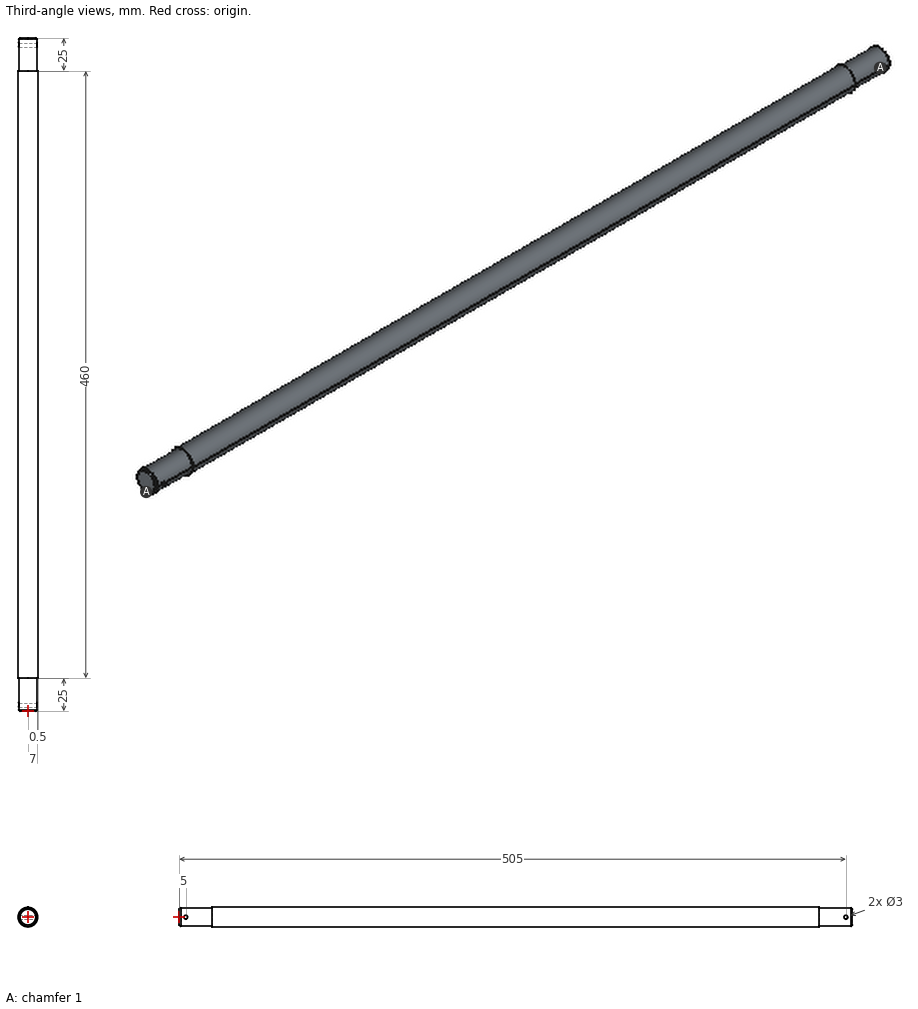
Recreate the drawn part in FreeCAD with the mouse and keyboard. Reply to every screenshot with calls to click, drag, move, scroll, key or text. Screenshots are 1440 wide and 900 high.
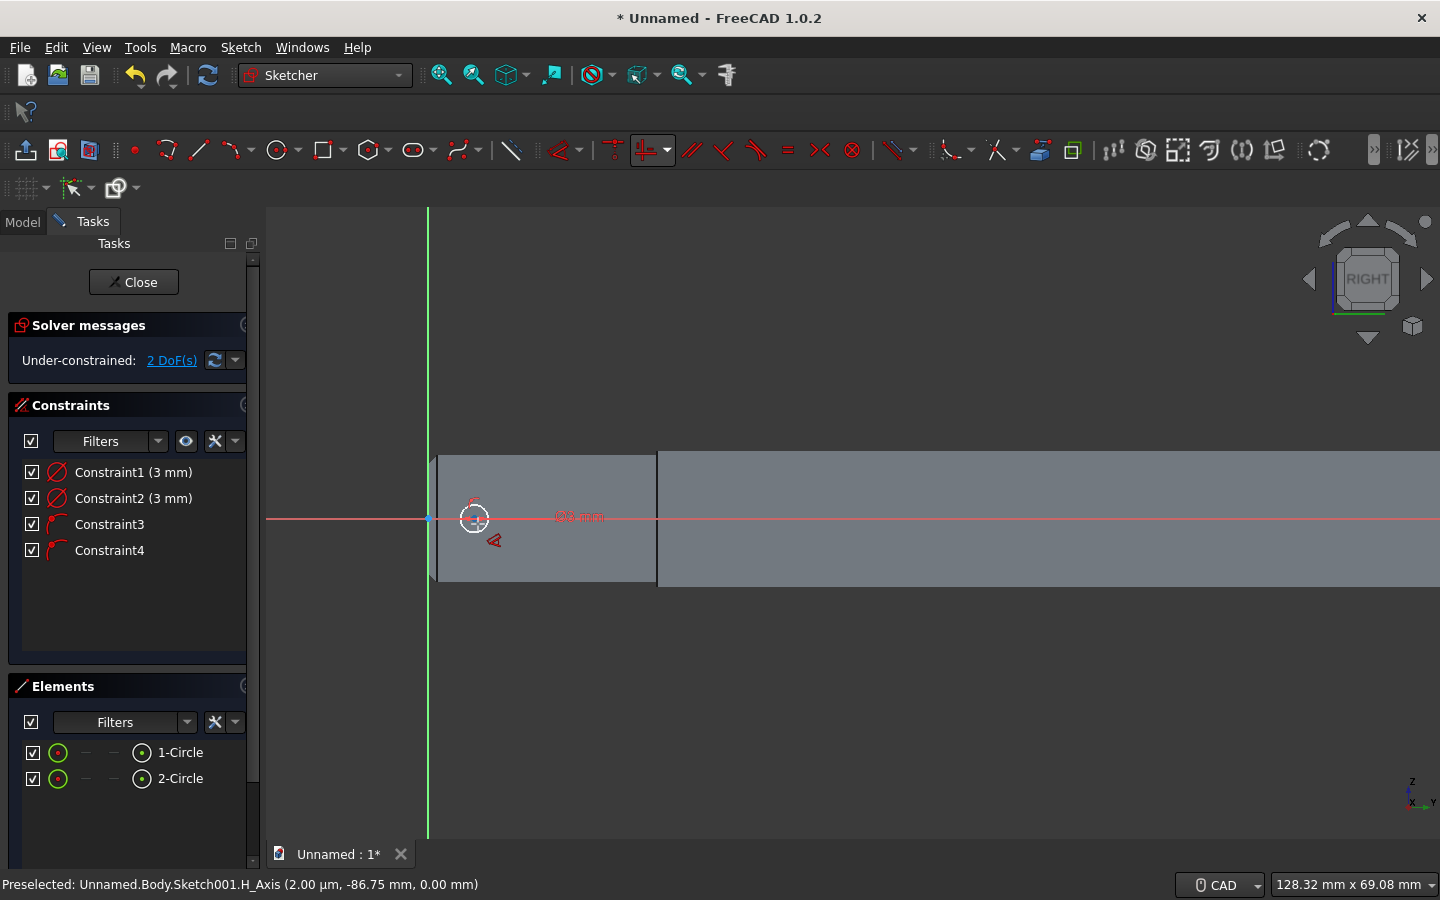
click(474, 519)
click(451, 553)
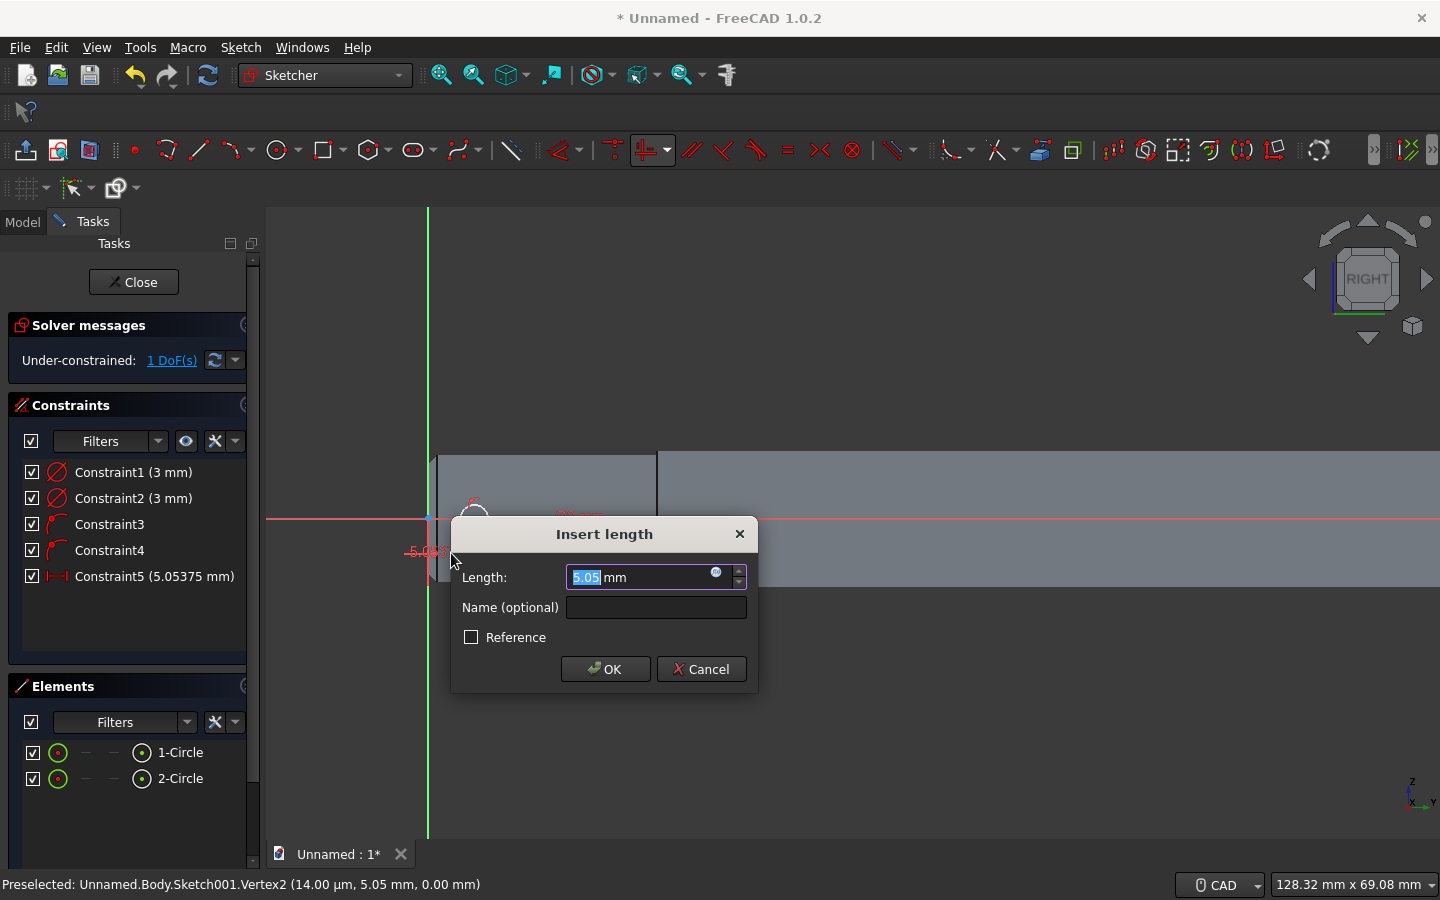
text(5)
key(Return)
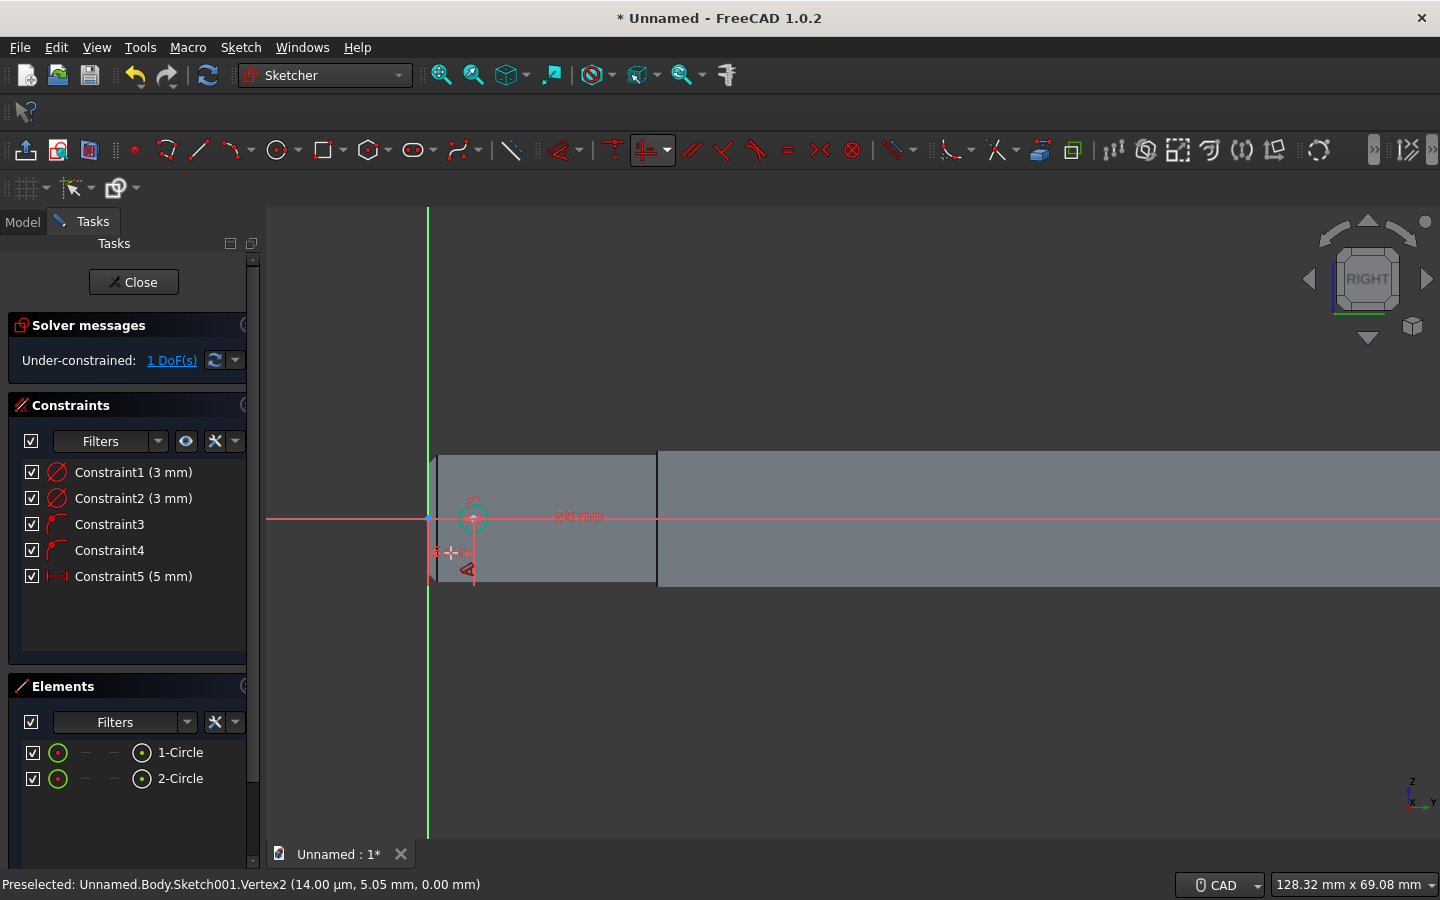
scroll(478, 524, down, 10)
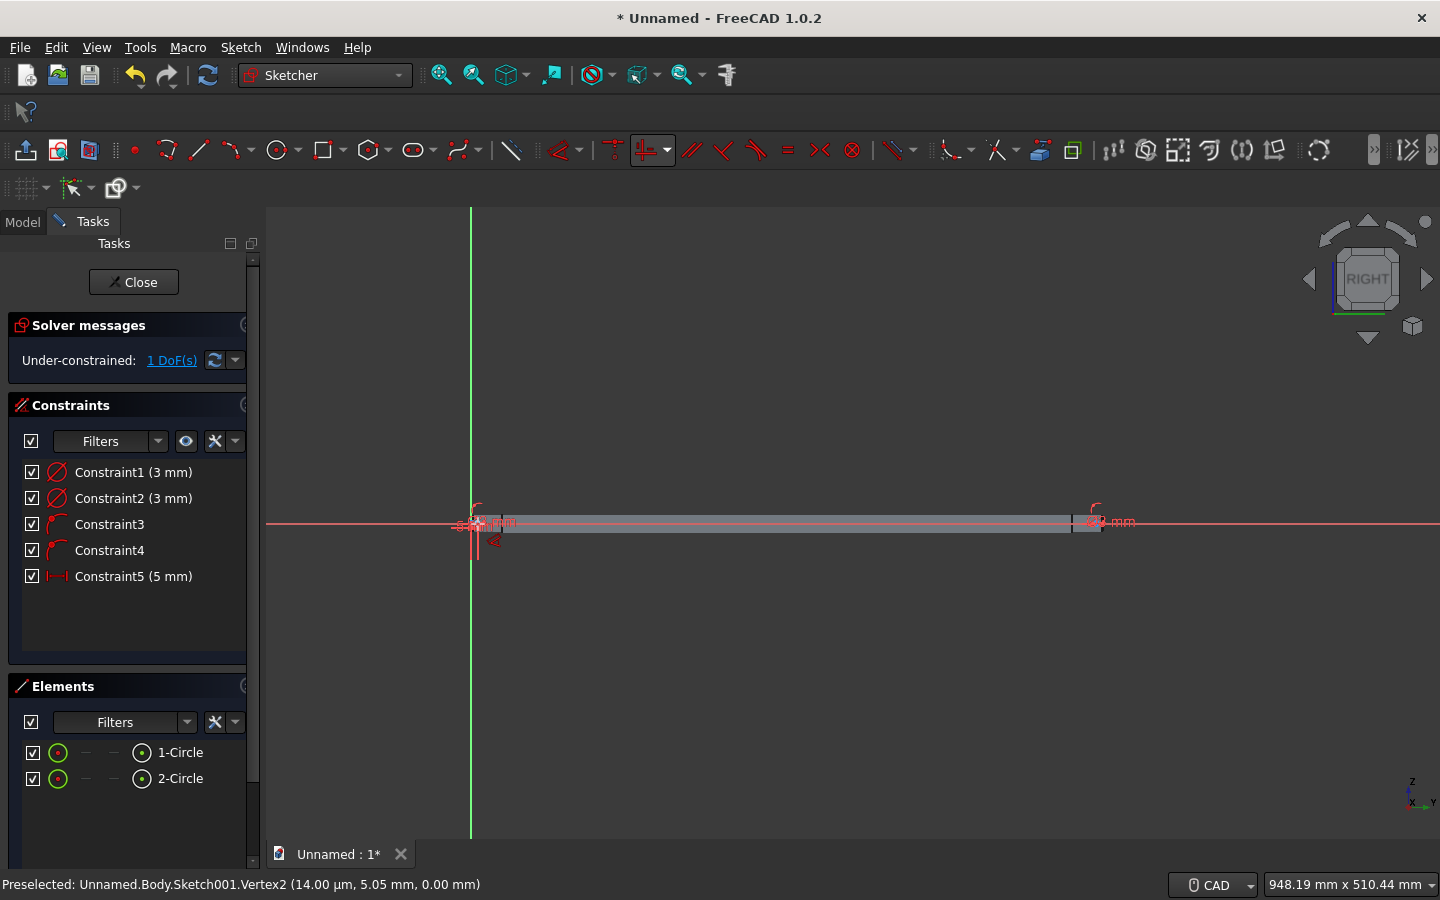
click(1097, 524)
click(784, 558)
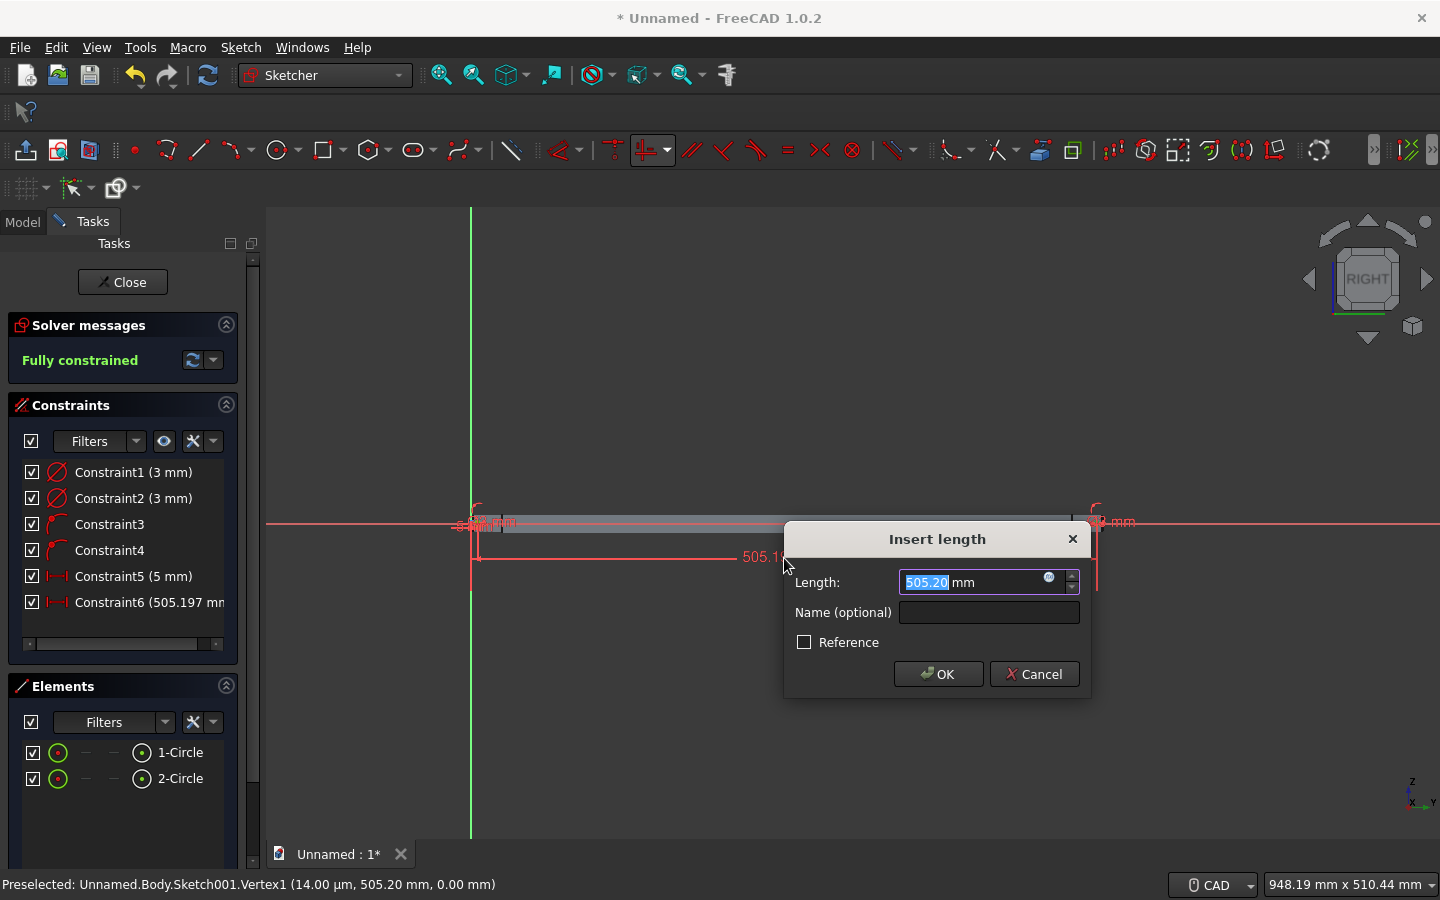
text(505)
key(Return)
key(Escape)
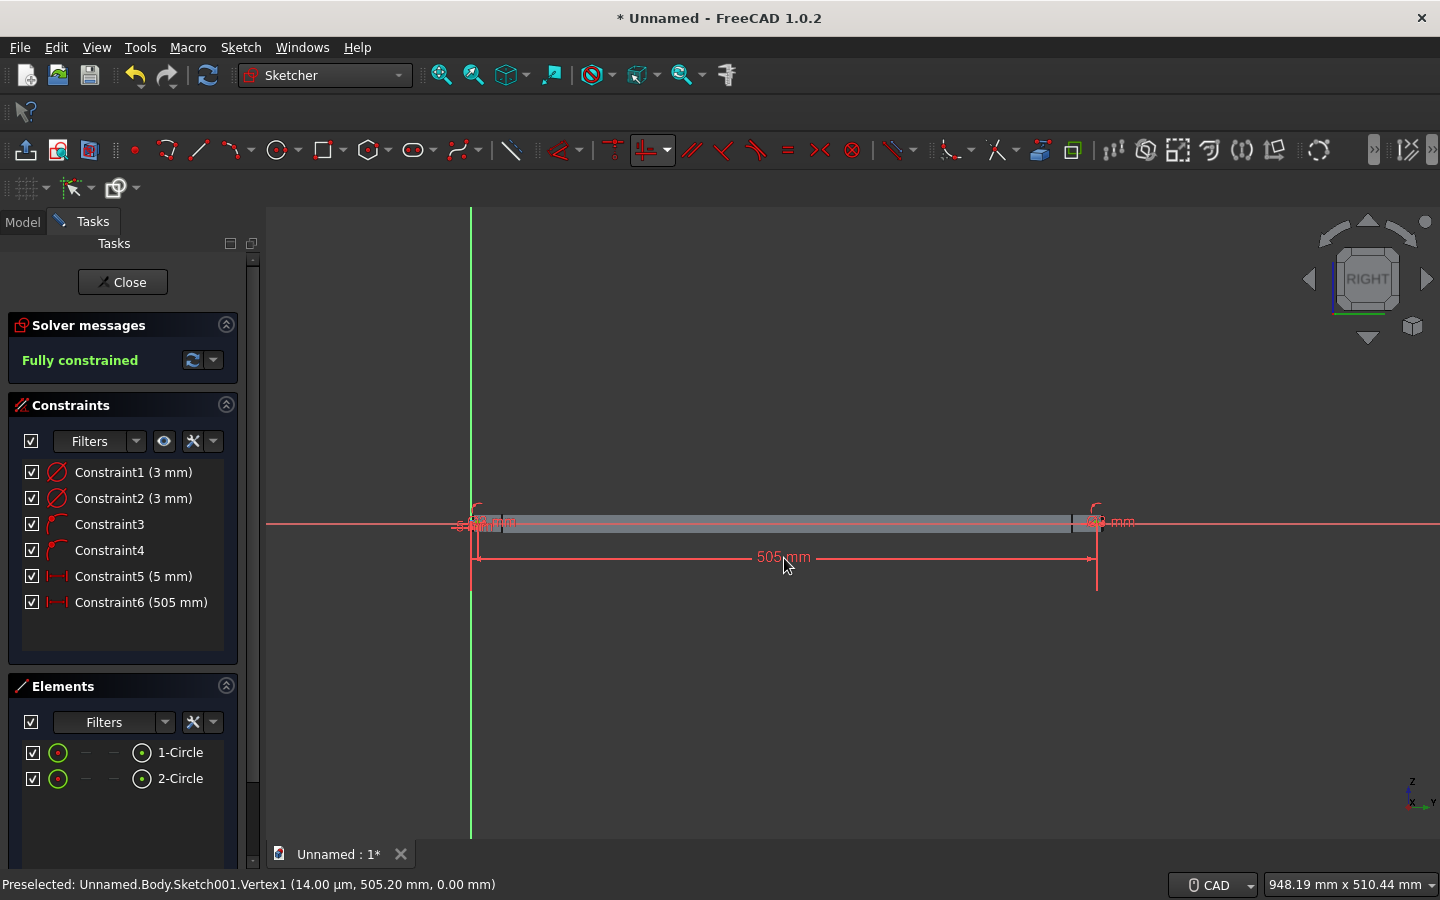
click(123, 282)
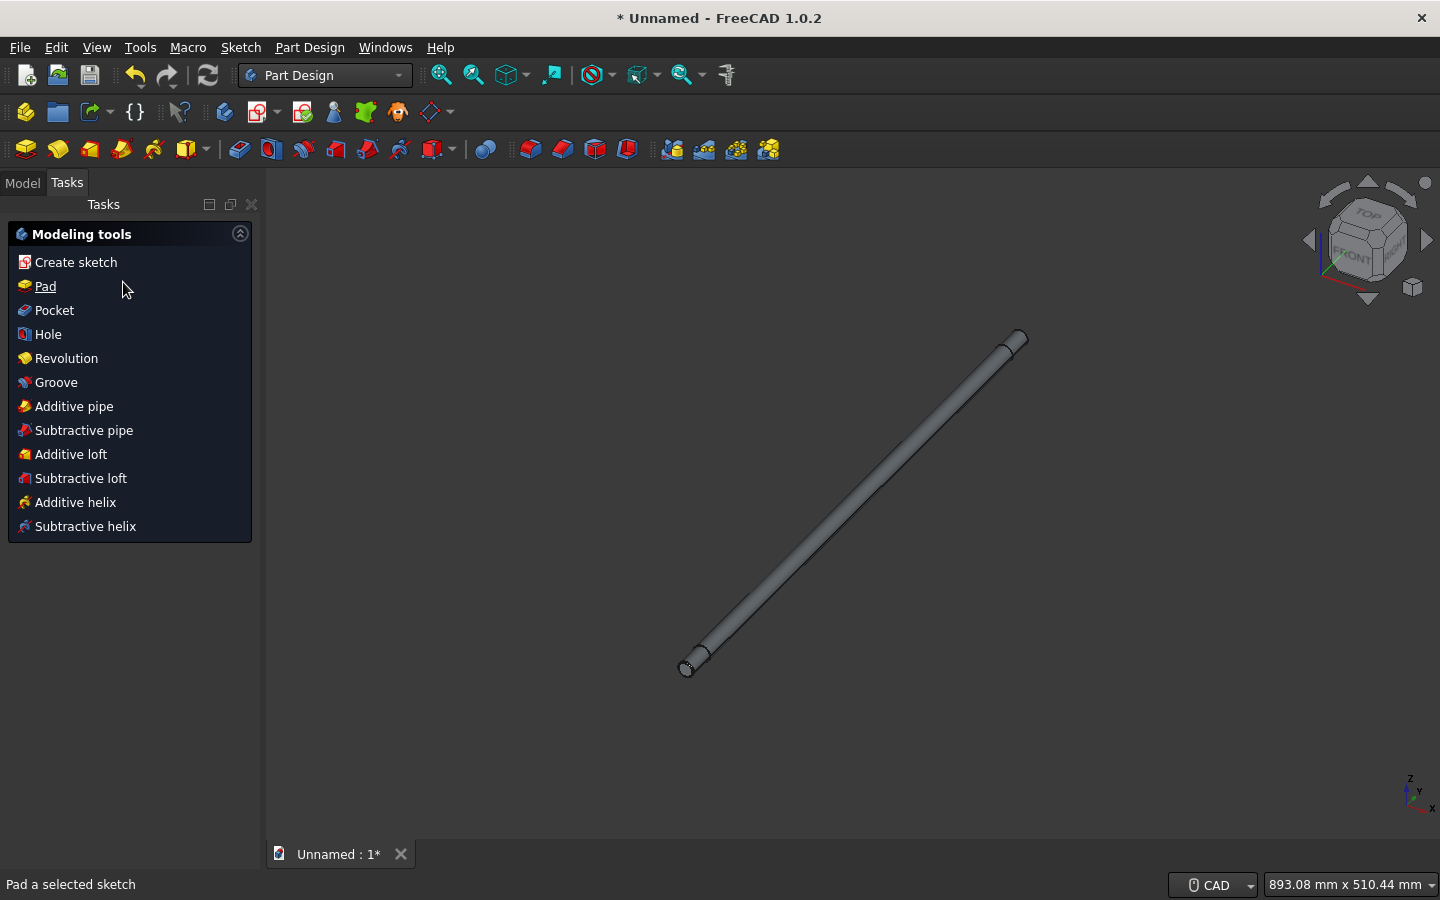
click(240, 150)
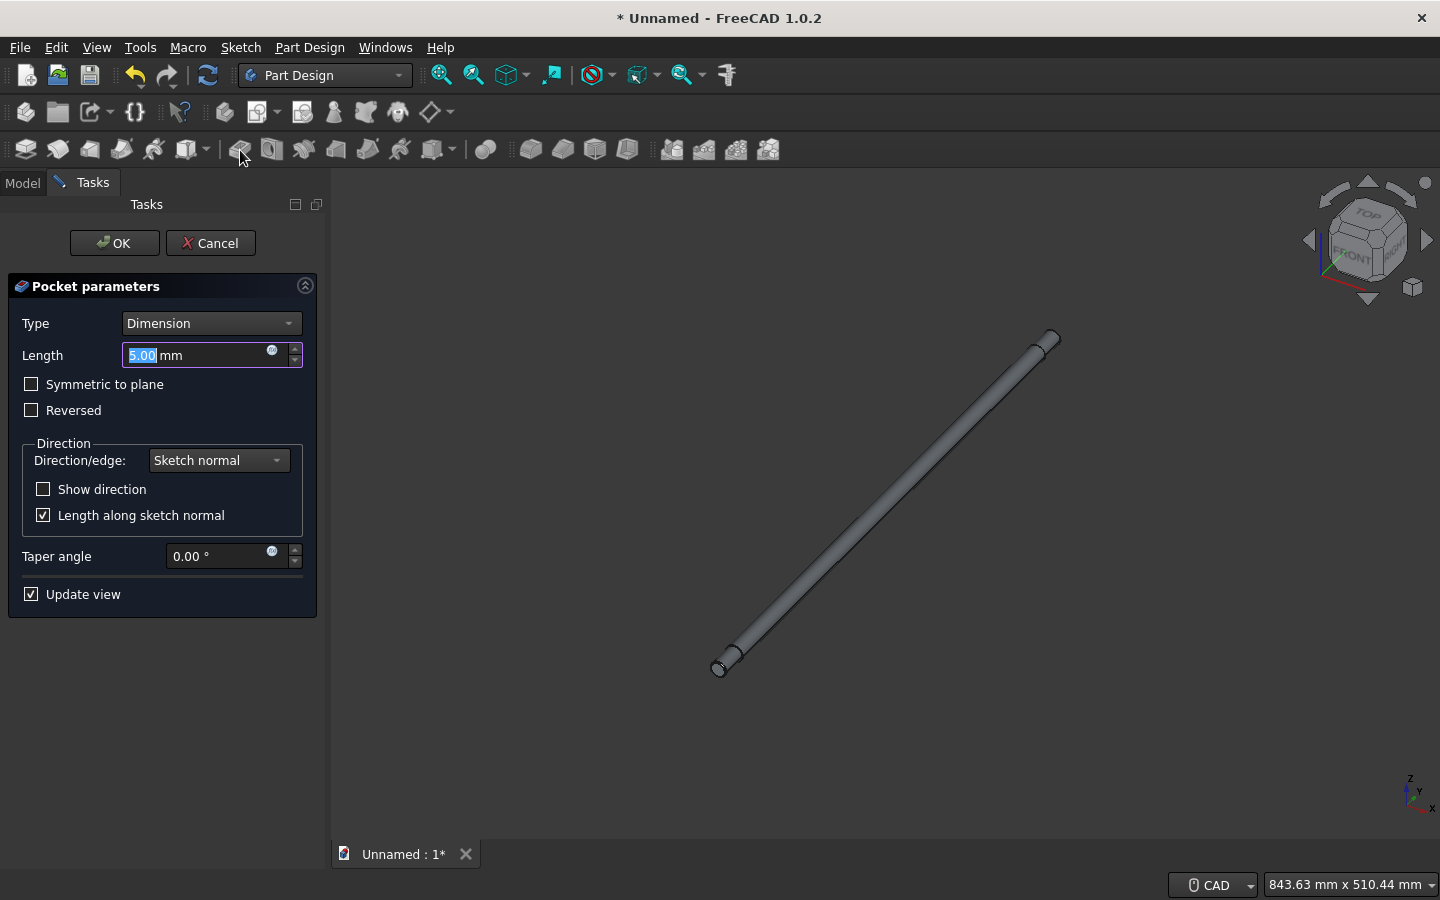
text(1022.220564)
key(Tab)